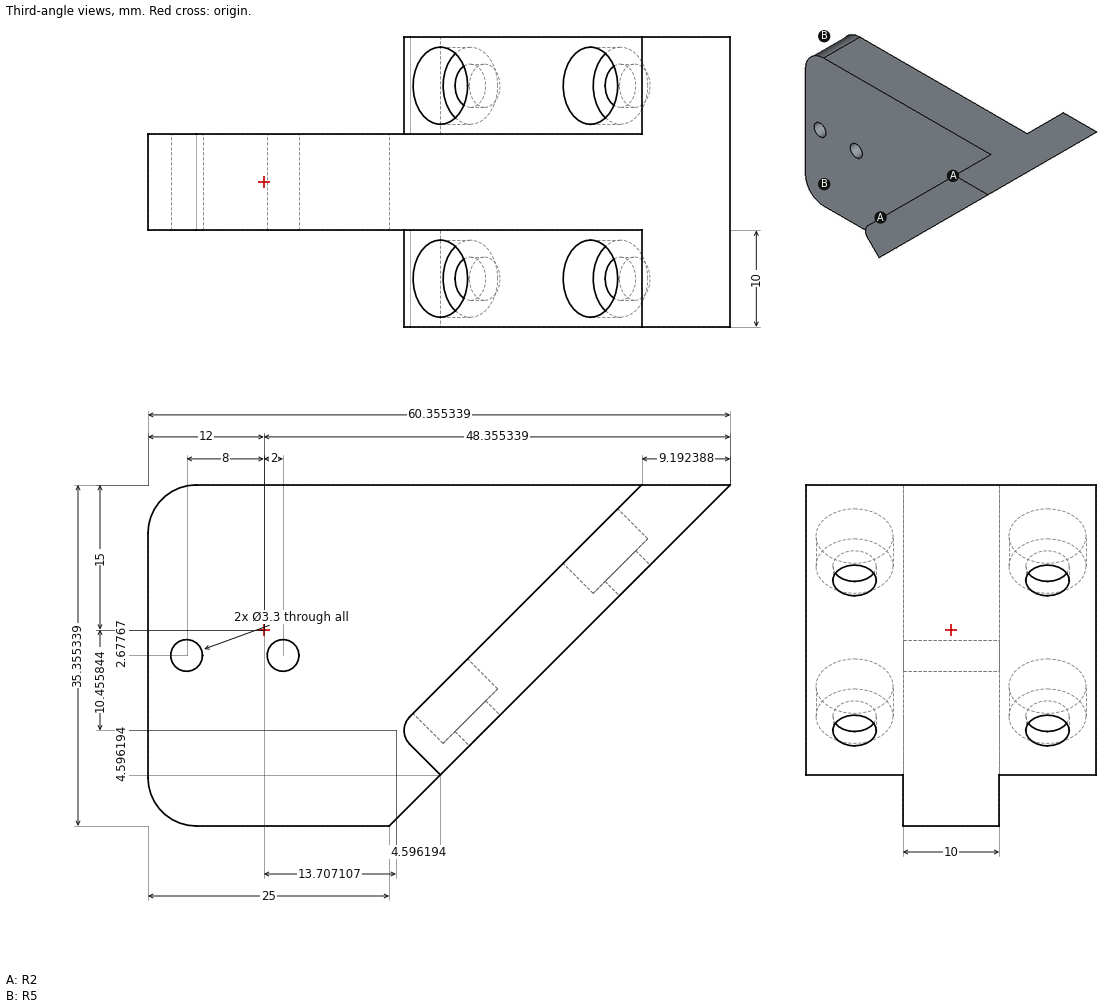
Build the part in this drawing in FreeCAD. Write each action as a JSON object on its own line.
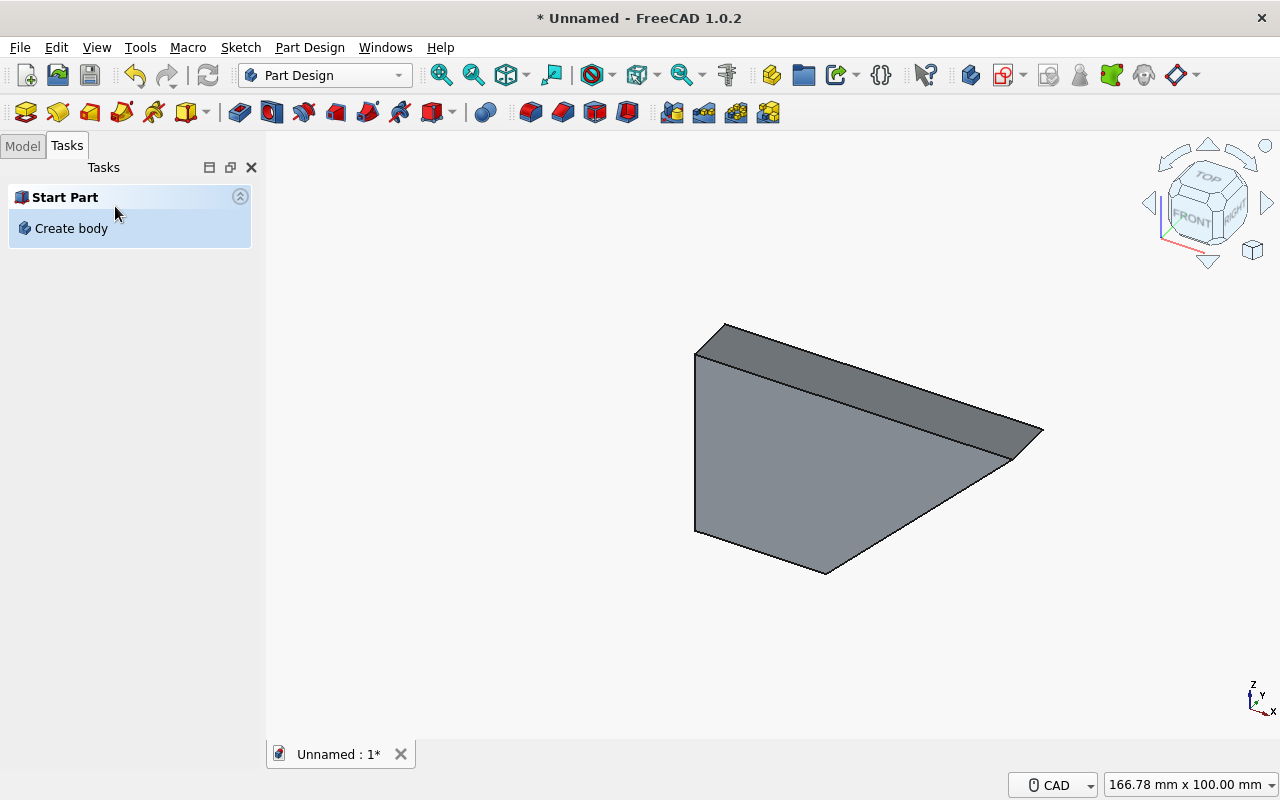
{"action": "left_click", "coordinate": [808, 479]}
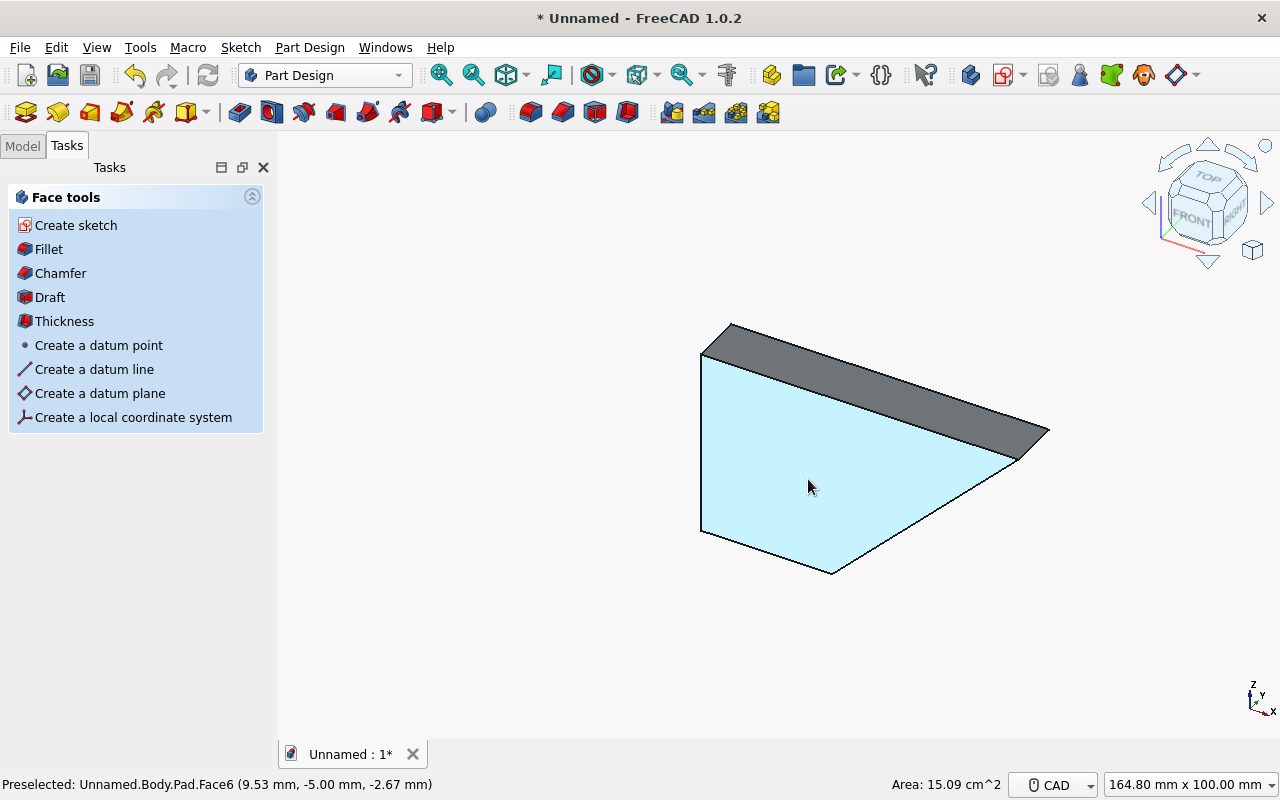
{"action": "left_click", "coordinate": [1004, 76]}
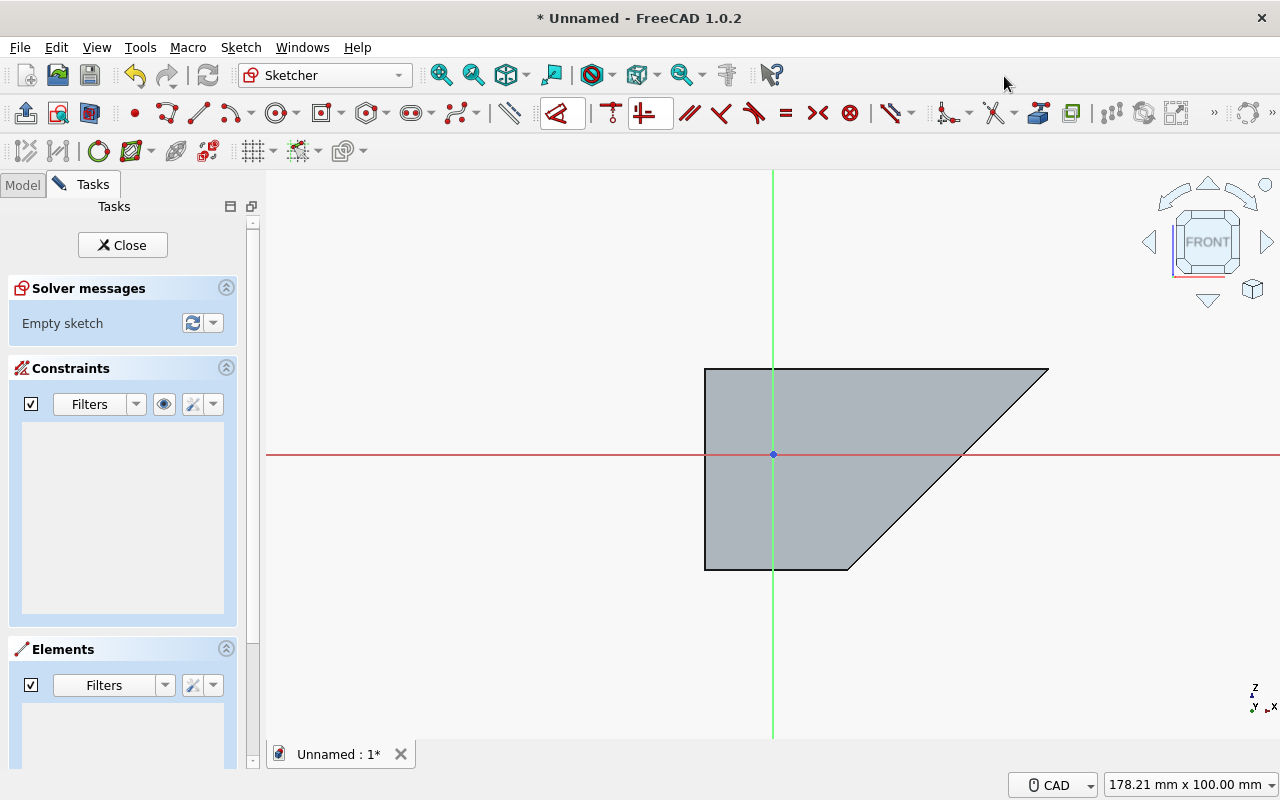
{"action": "scroll", "coordinate": [764, 469], "scroll_direction": "up", "scroll_amount": 10}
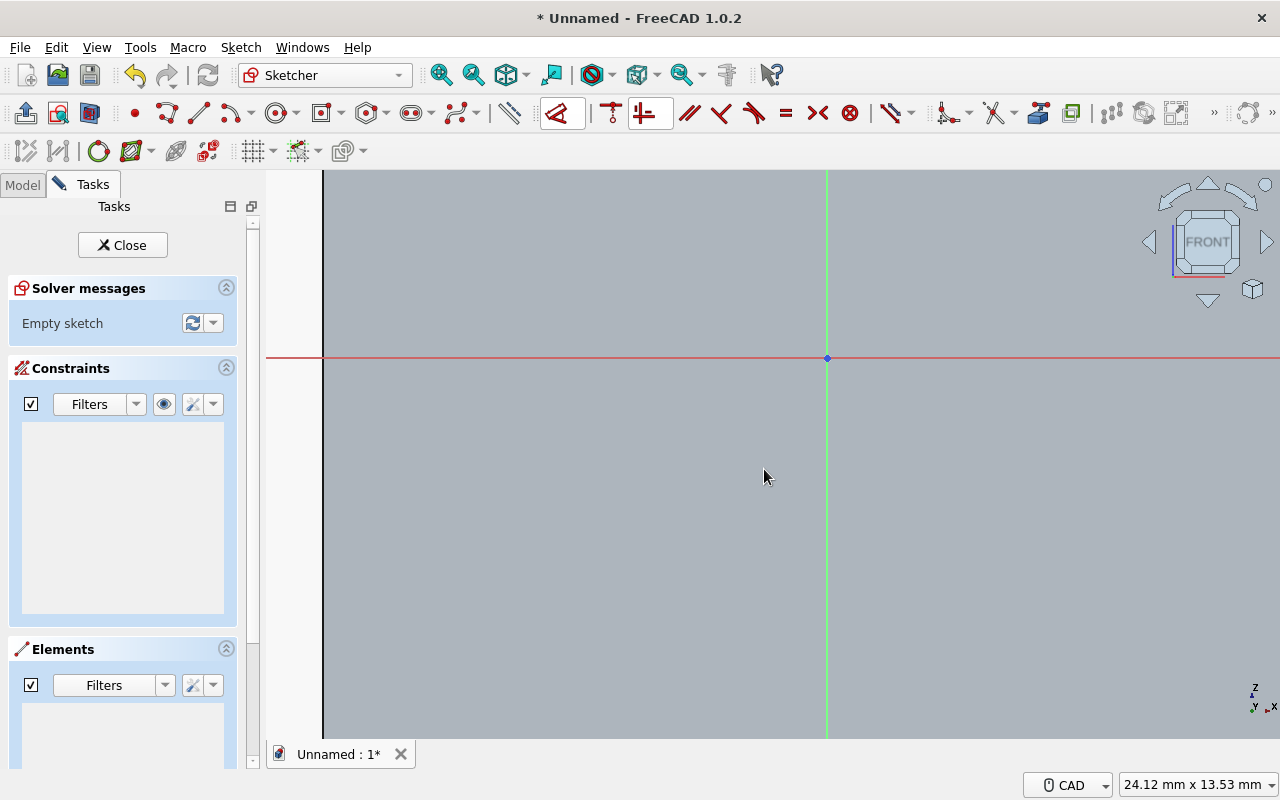
{"action": "left_click", "coordinate": [276, 114]}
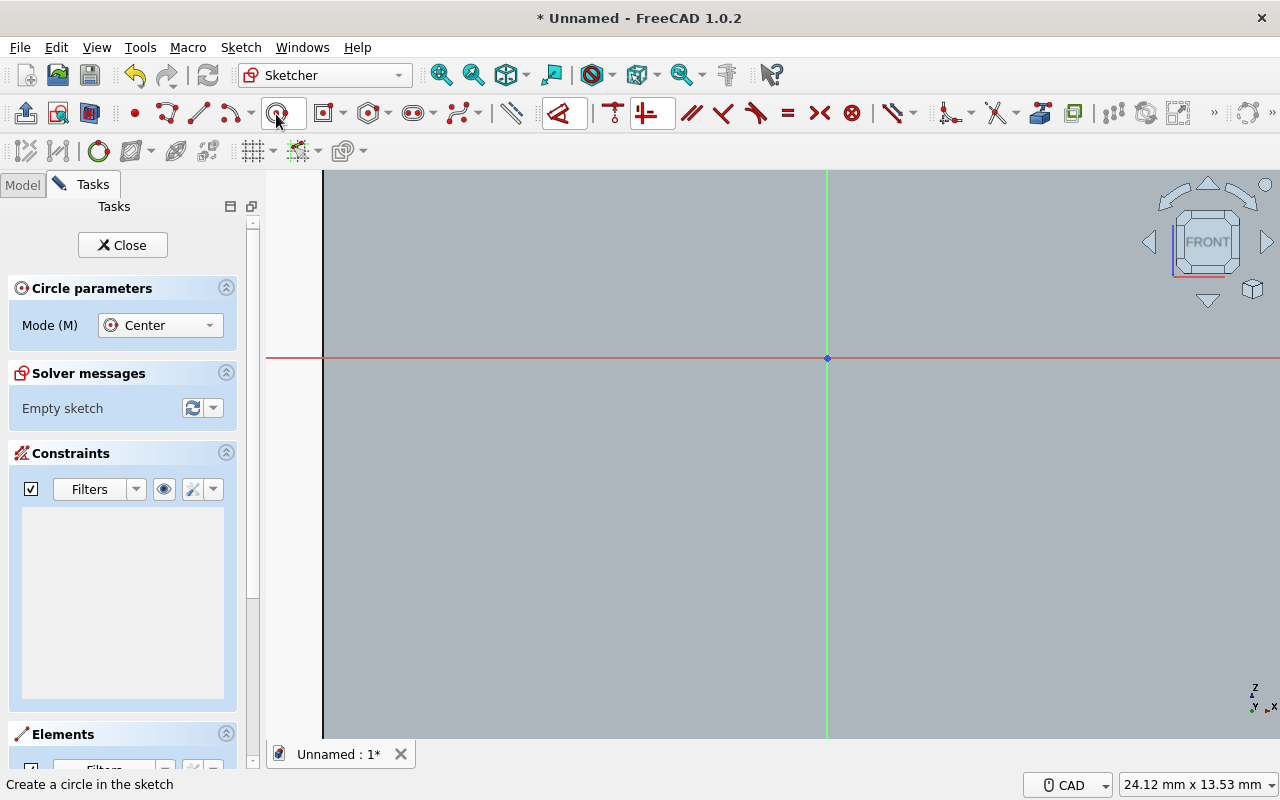
{"action": "left_click", "coordinate": [491, 471]}
{"action": "left_click", "coordinate": [540, 422]}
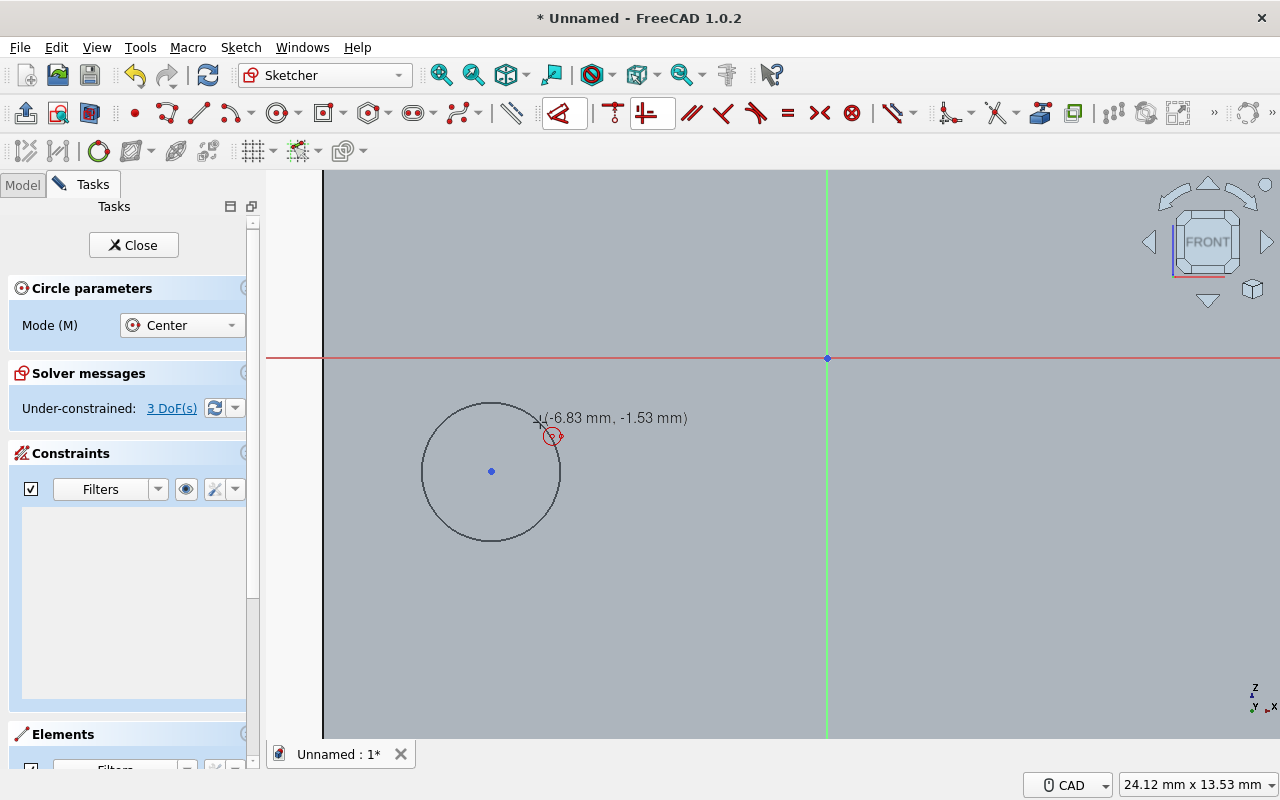
{"action": "left_click", "coordinate": [911, 471]}
{"action": "left_click", "coordinate": [961, 422]}
{"action": "key", "text": "Escape"}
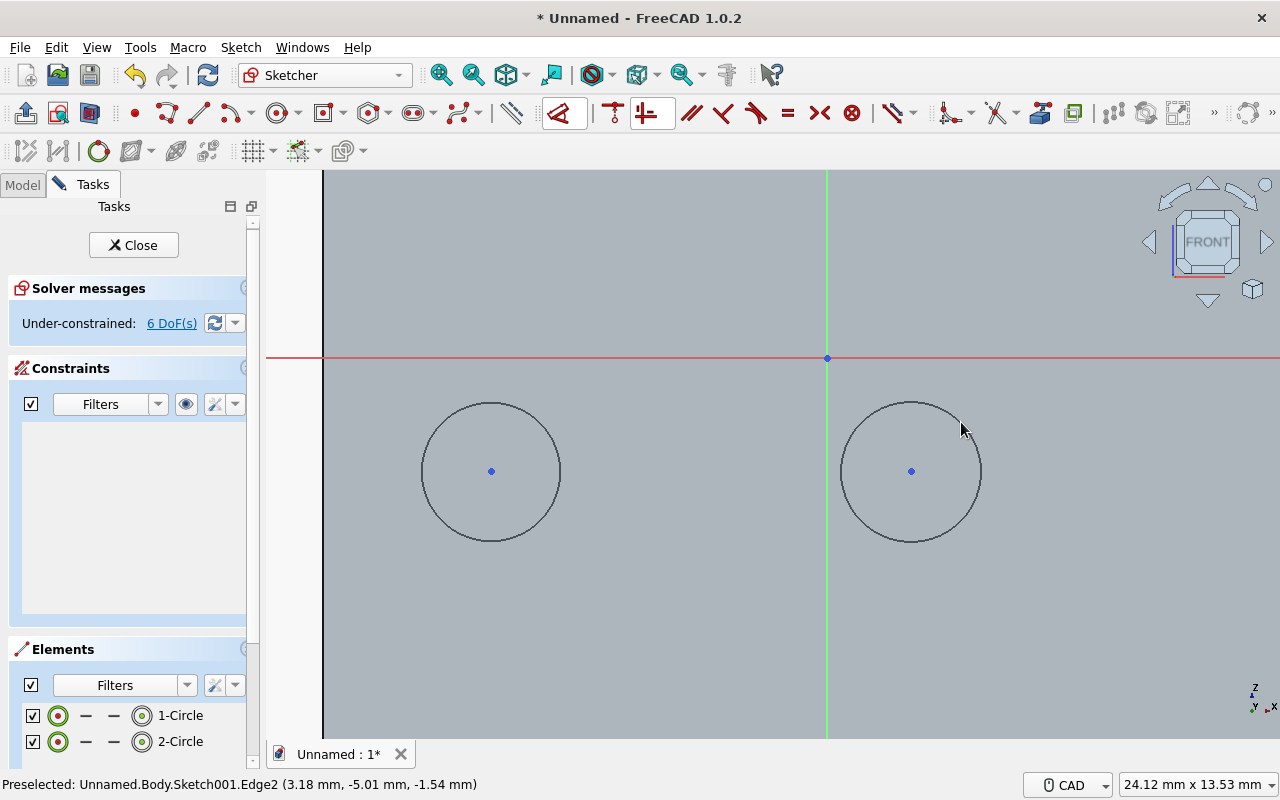
{"action": "left_click", "coordinate": [540, 423]}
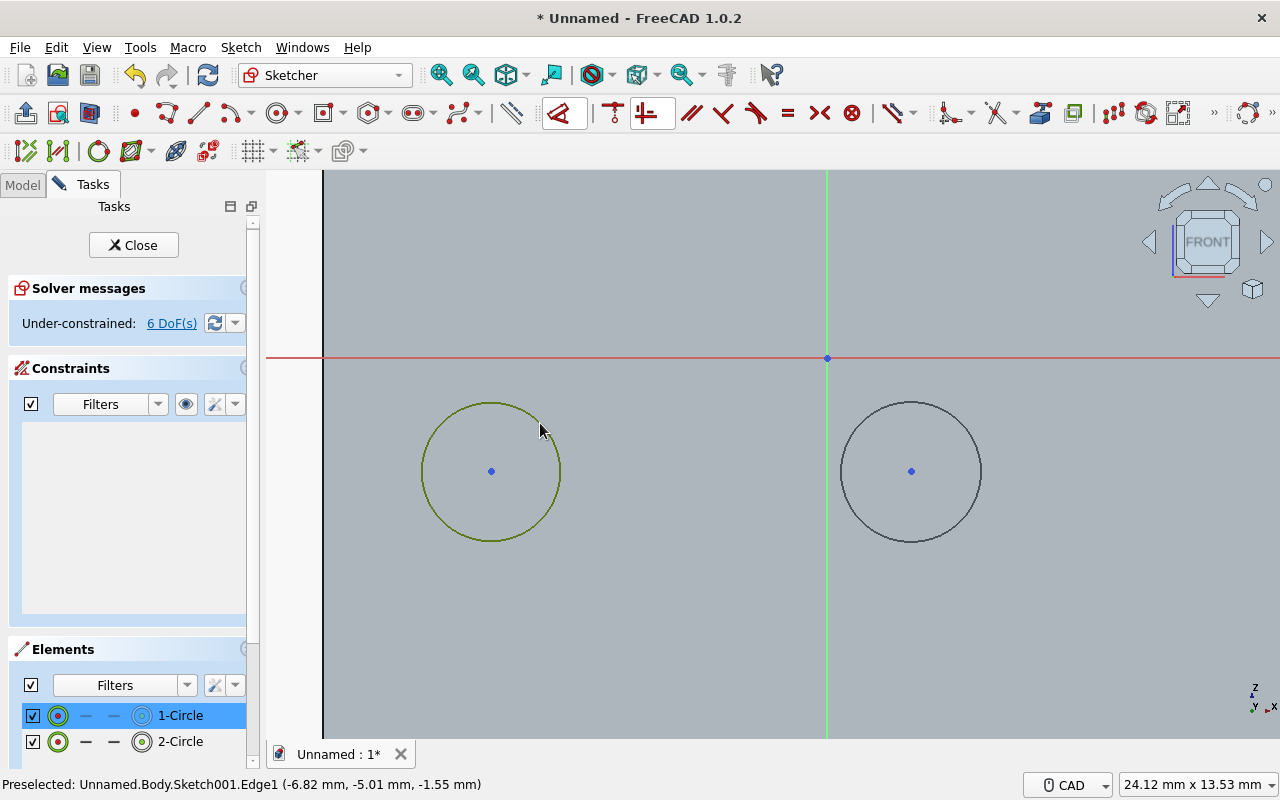
{"action": "left_click", "coordinate": [960, 422]}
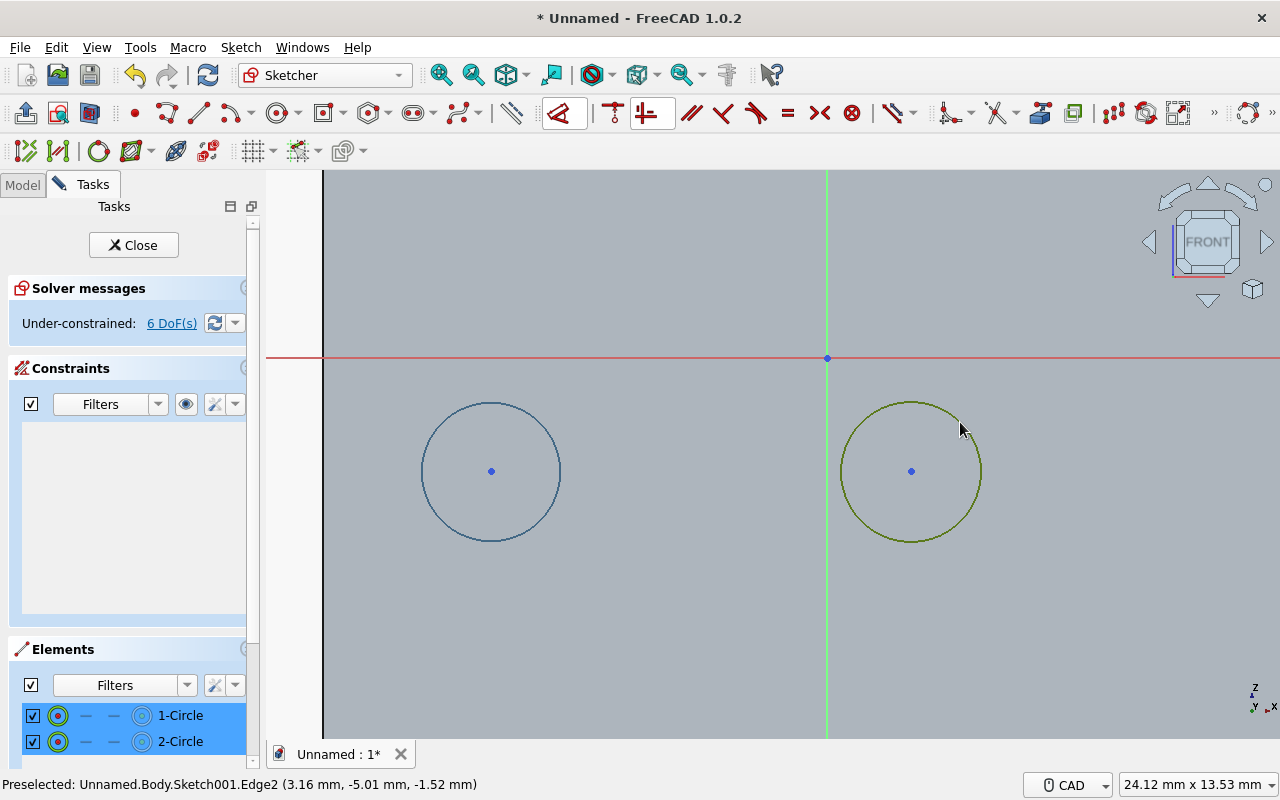
{"action": "left_click", "coordinate": [788, 114]}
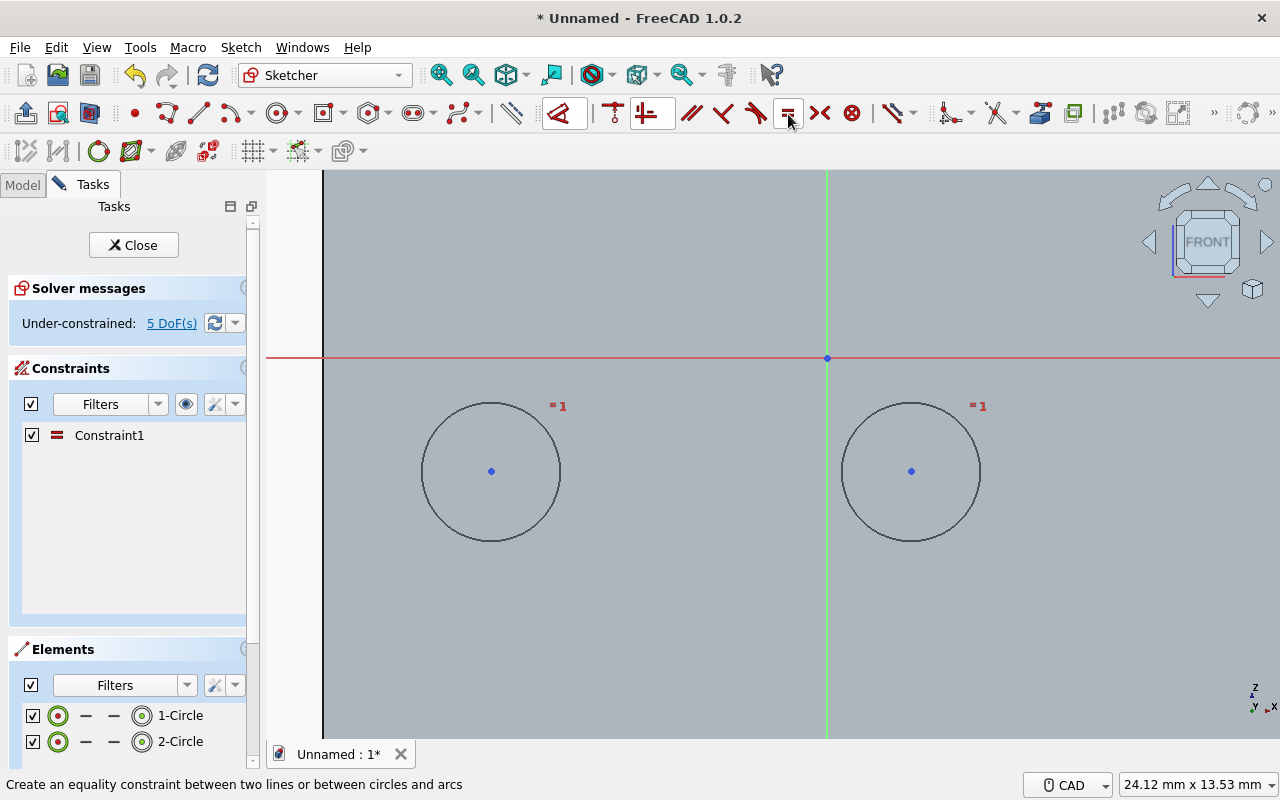
{"action": "left_click", "coordinate": [491, 472]}